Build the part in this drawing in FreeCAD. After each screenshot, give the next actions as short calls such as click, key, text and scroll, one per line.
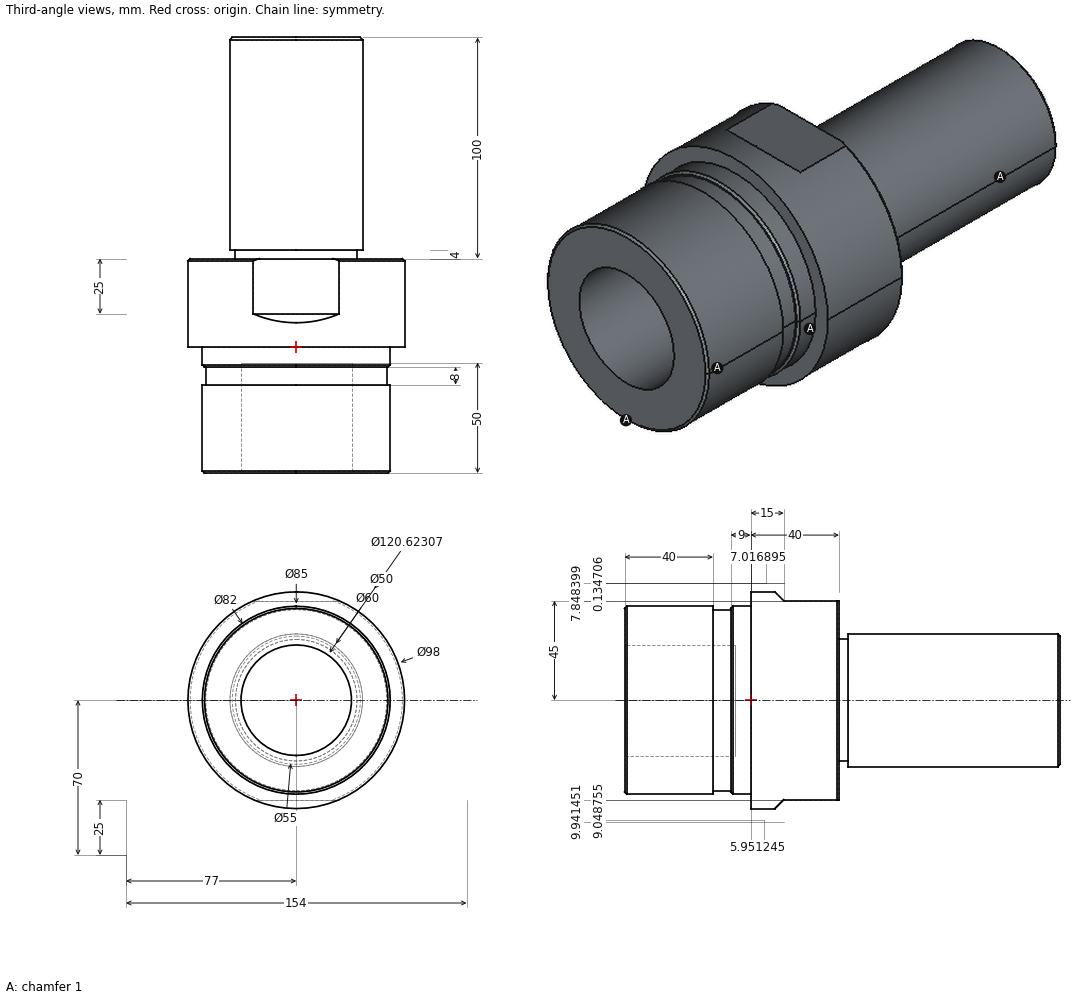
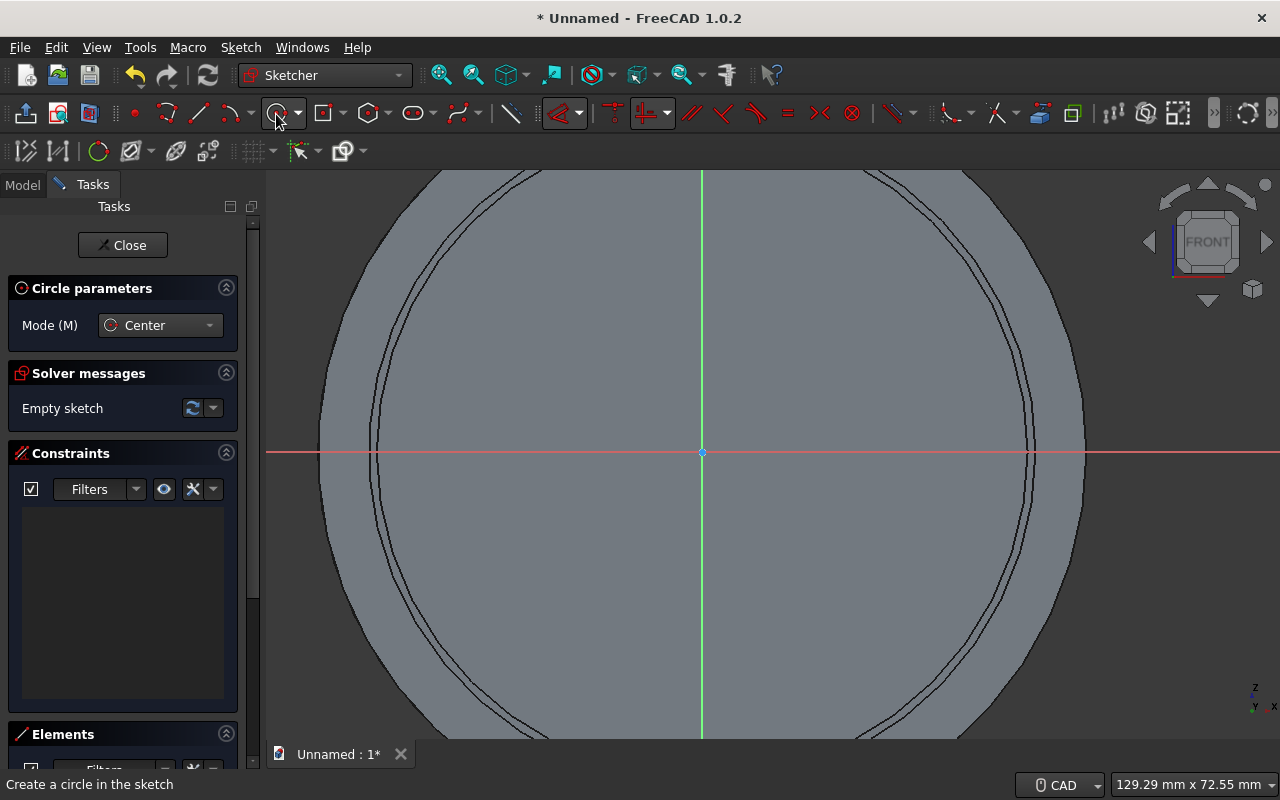
click(702, 452)
click(841, 314)
key(Escape)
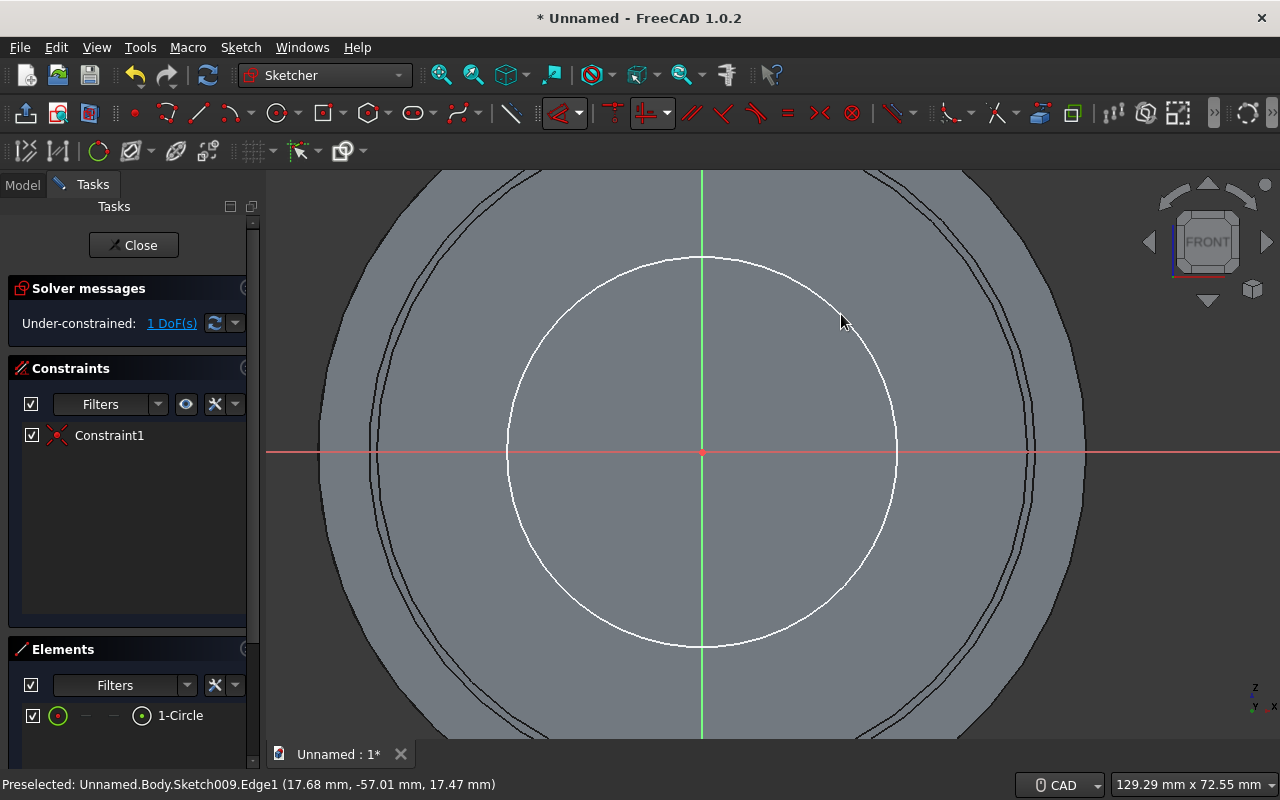
click(840, 314)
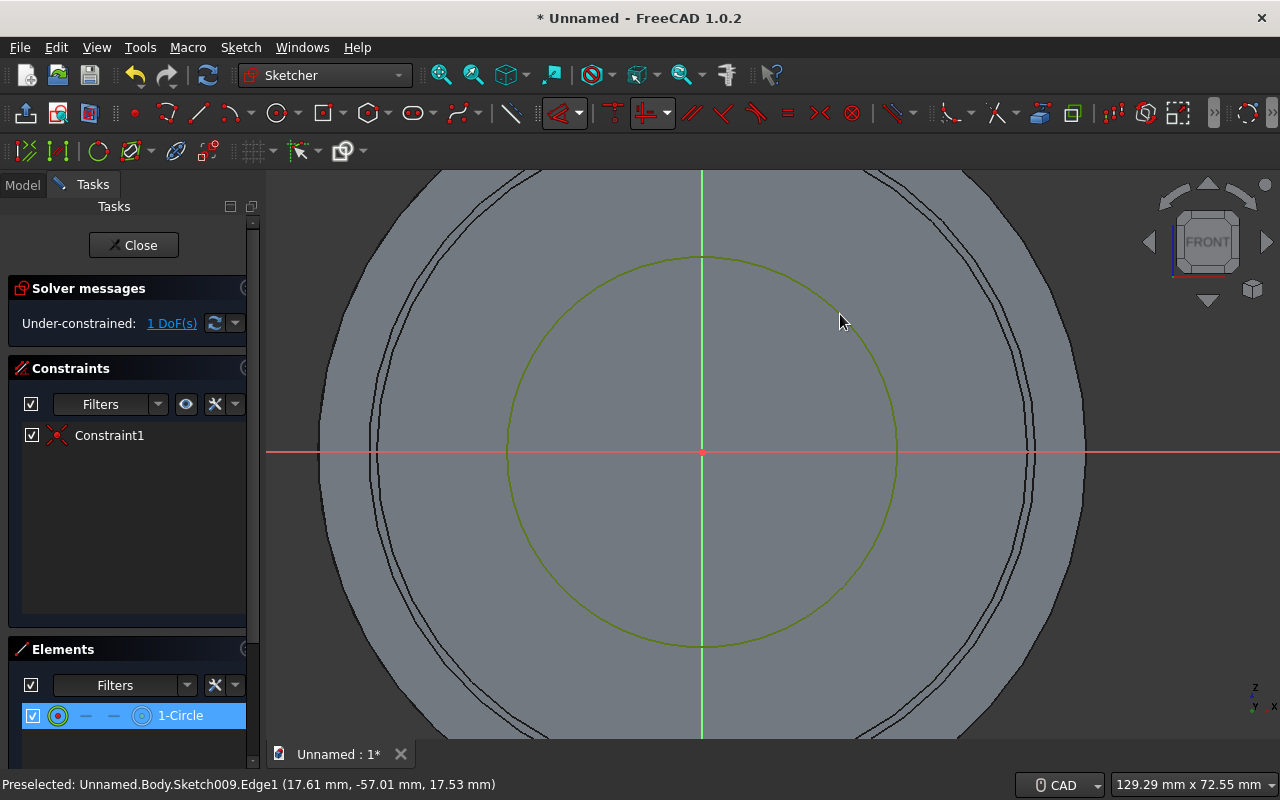
click(582, 114)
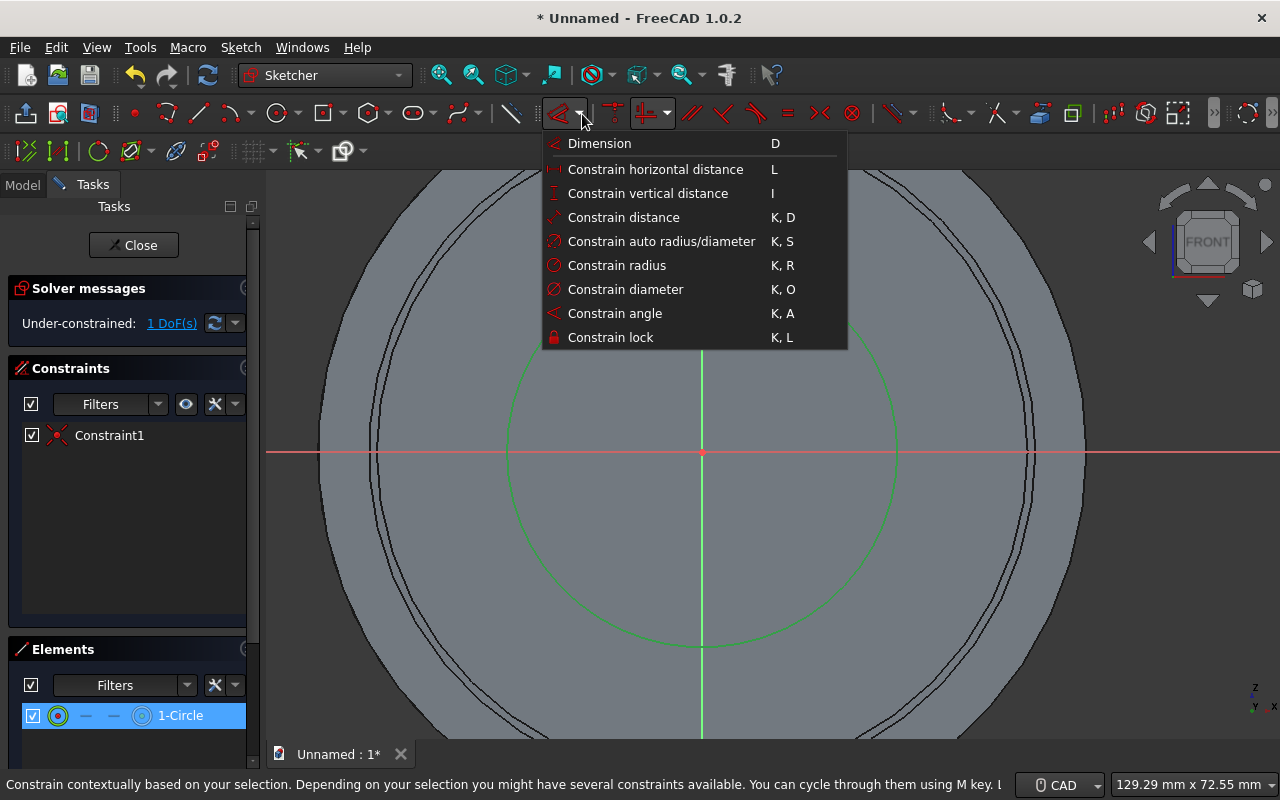
click(695, 289)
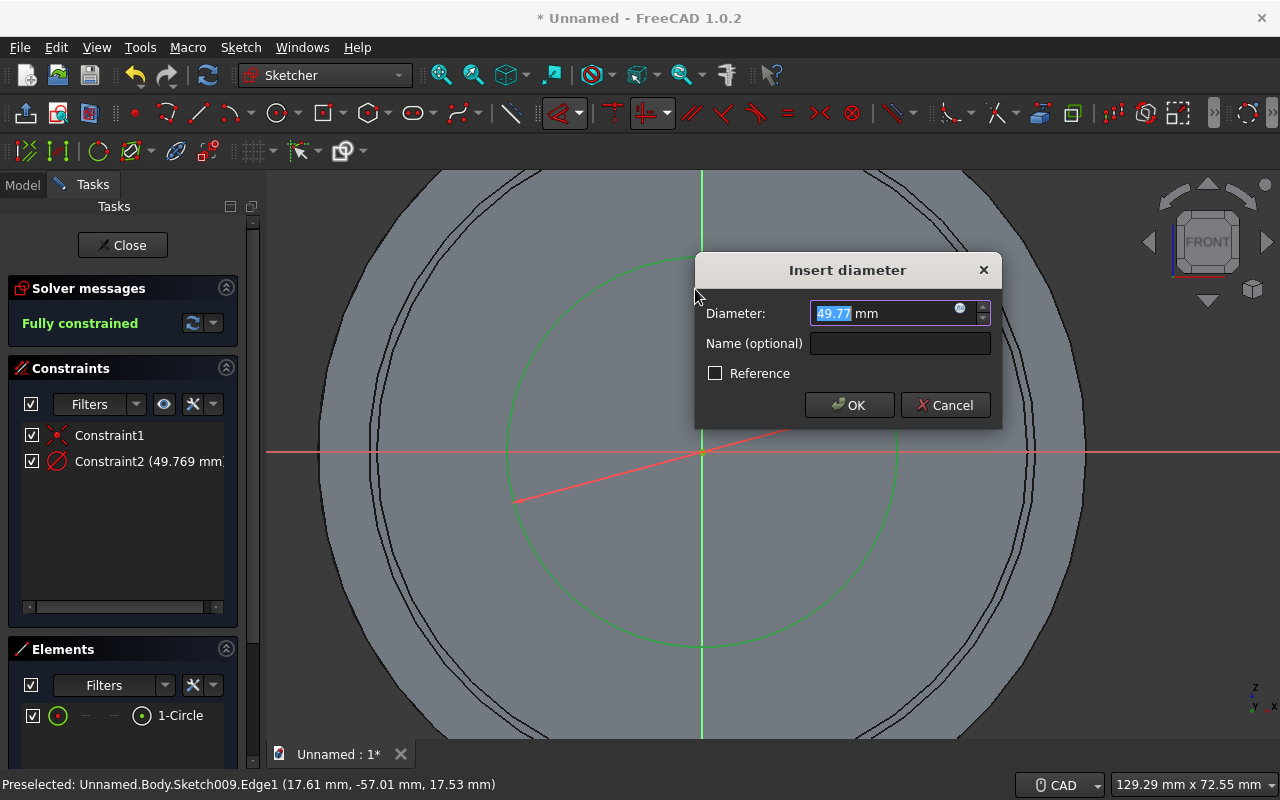
text(50)
key(Return)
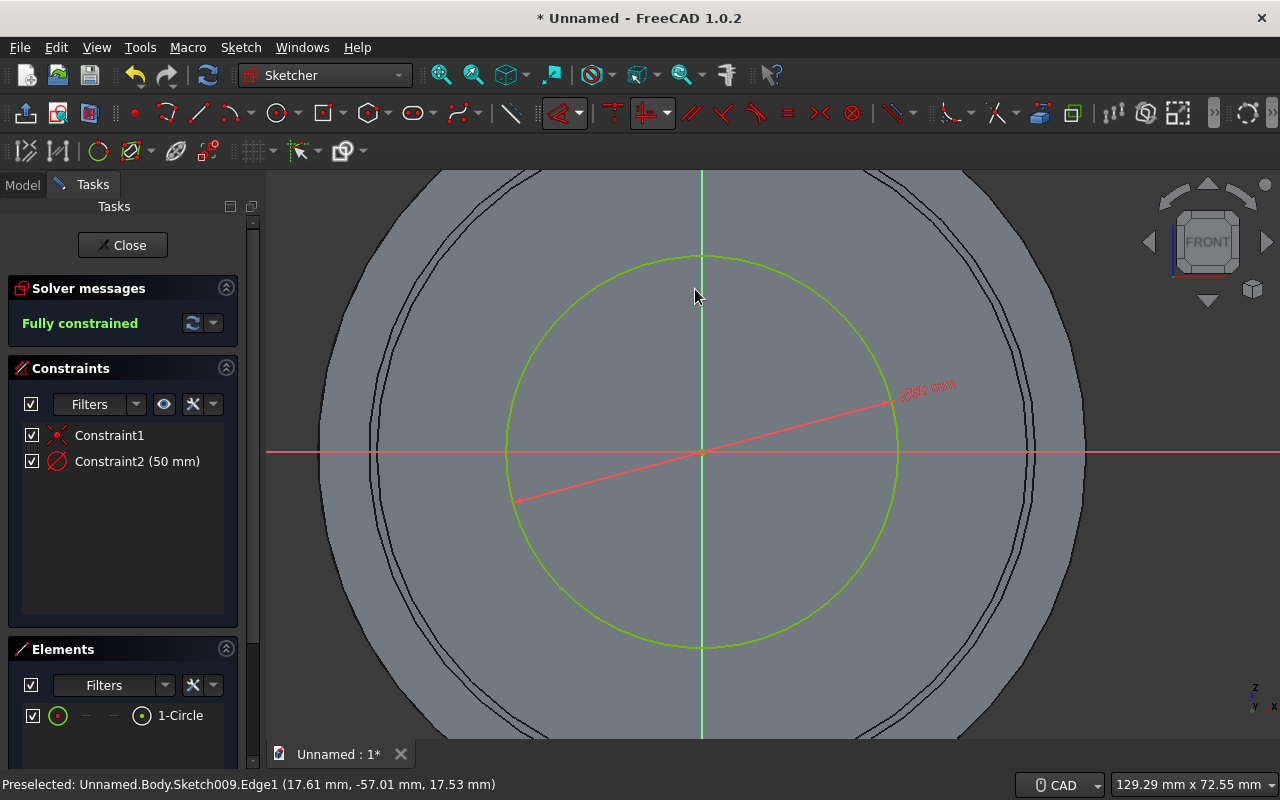
click(123, 245)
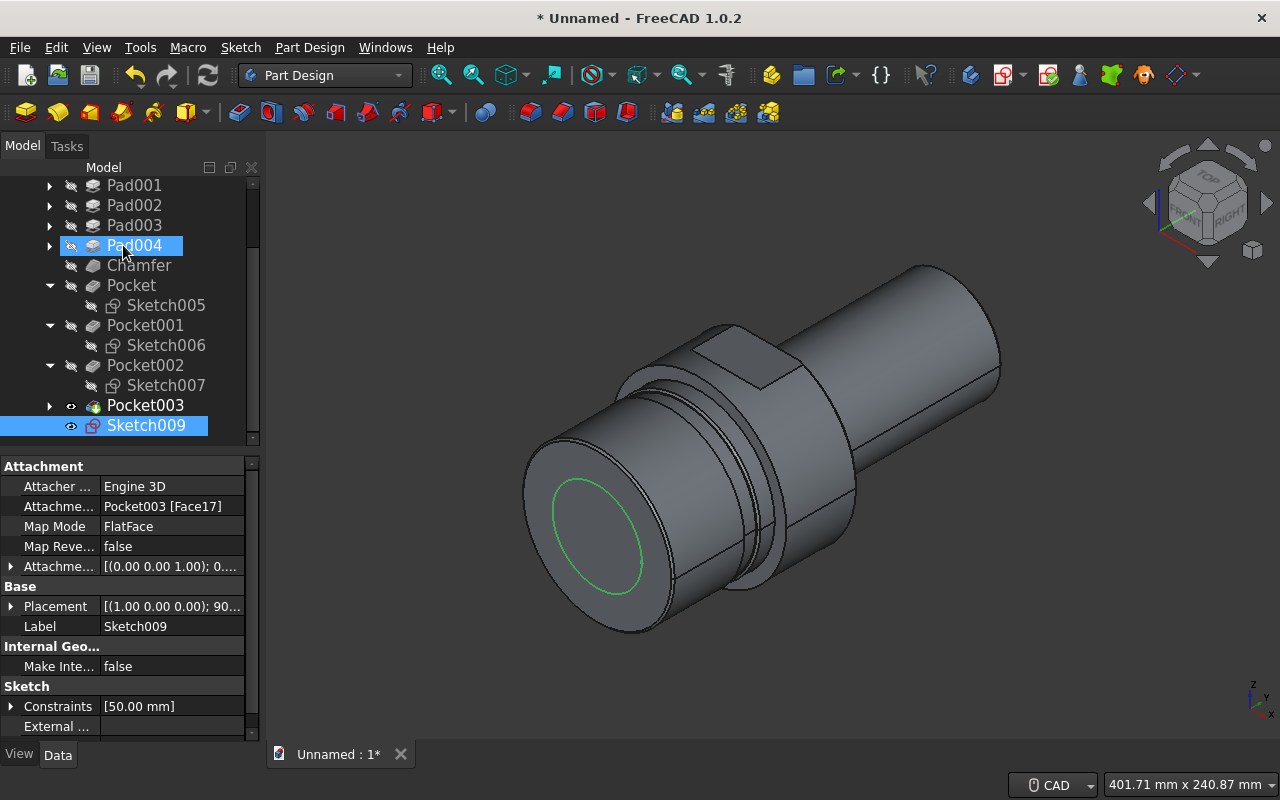
click(240, 112)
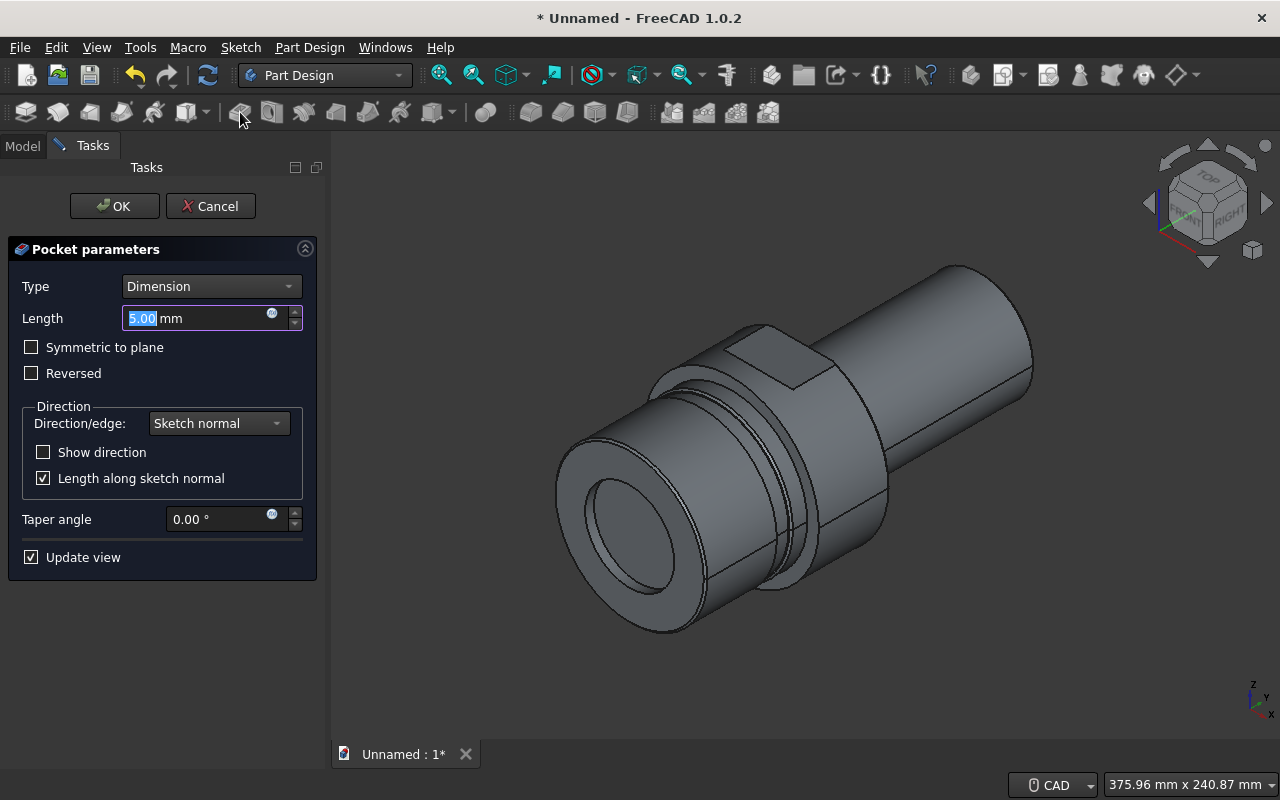
text(50)
key(Tab)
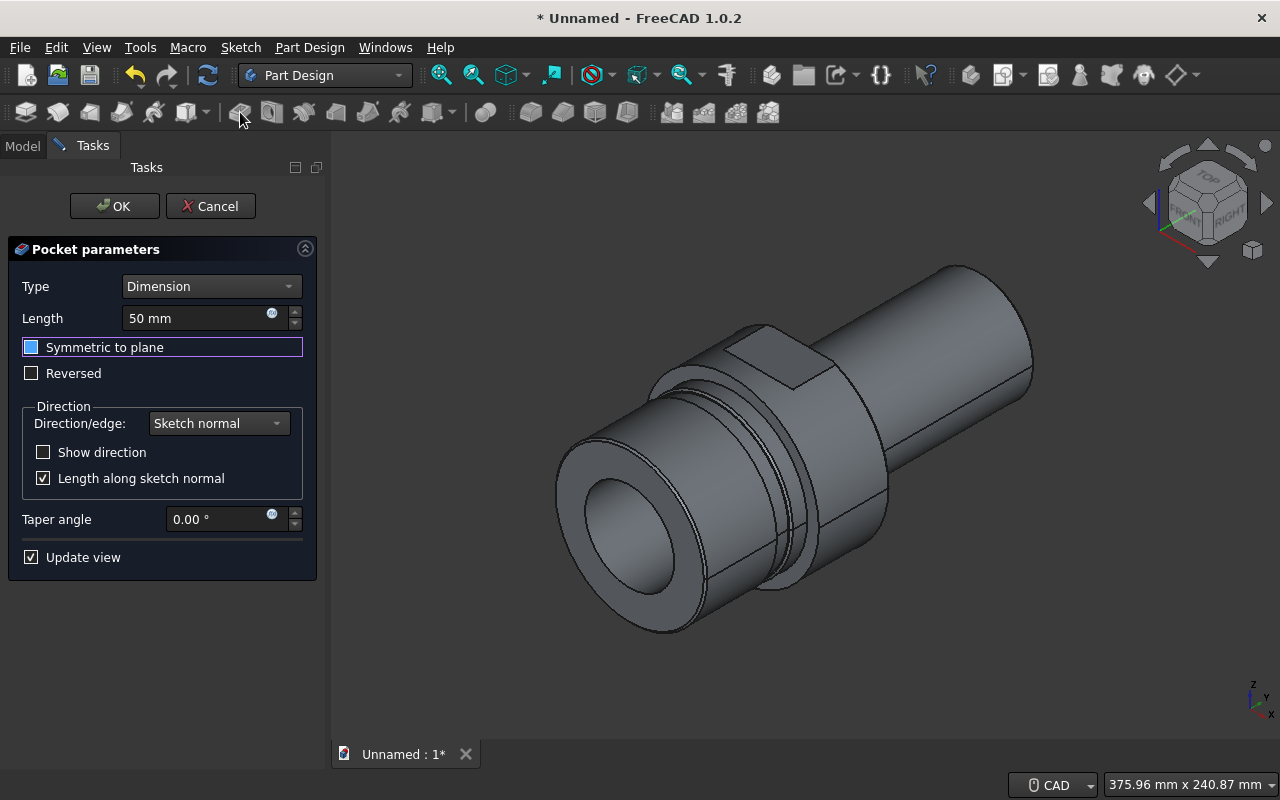
click(115, 206)